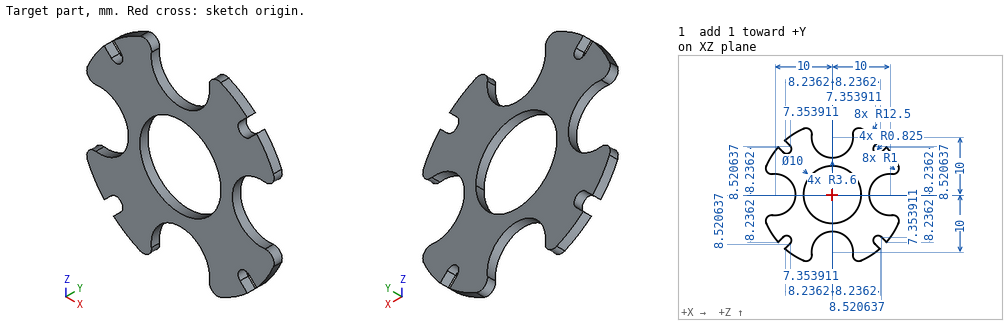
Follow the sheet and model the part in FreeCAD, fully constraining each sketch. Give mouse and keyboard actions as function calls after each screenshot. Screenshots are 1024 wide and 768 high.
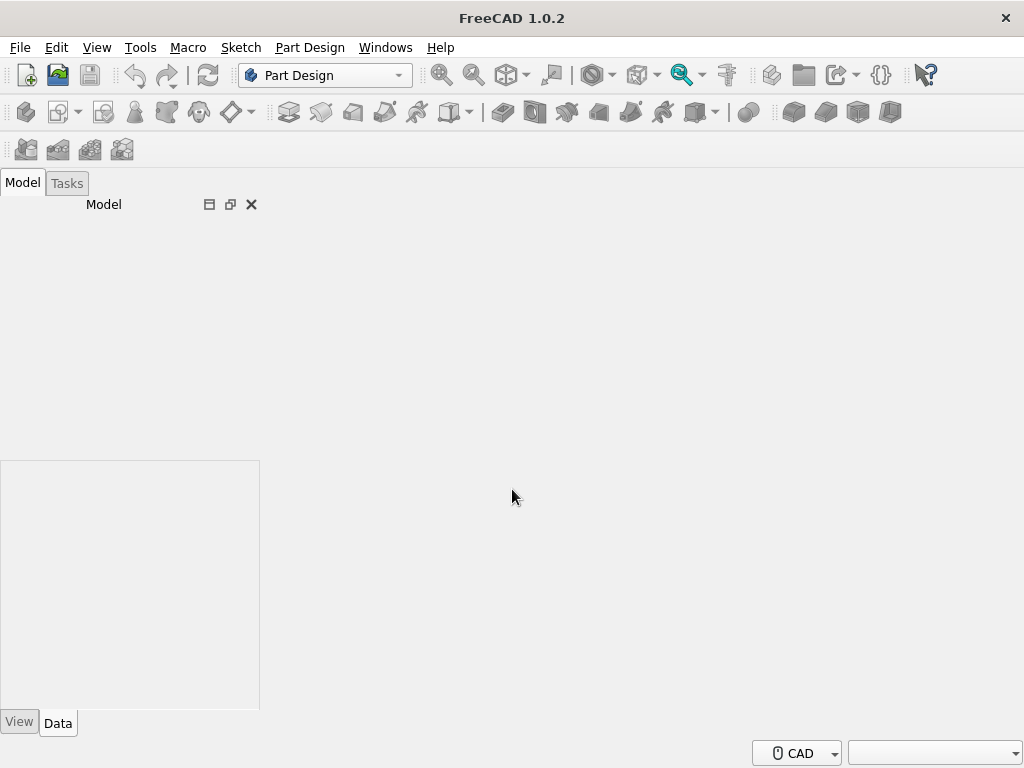
click(26, 76)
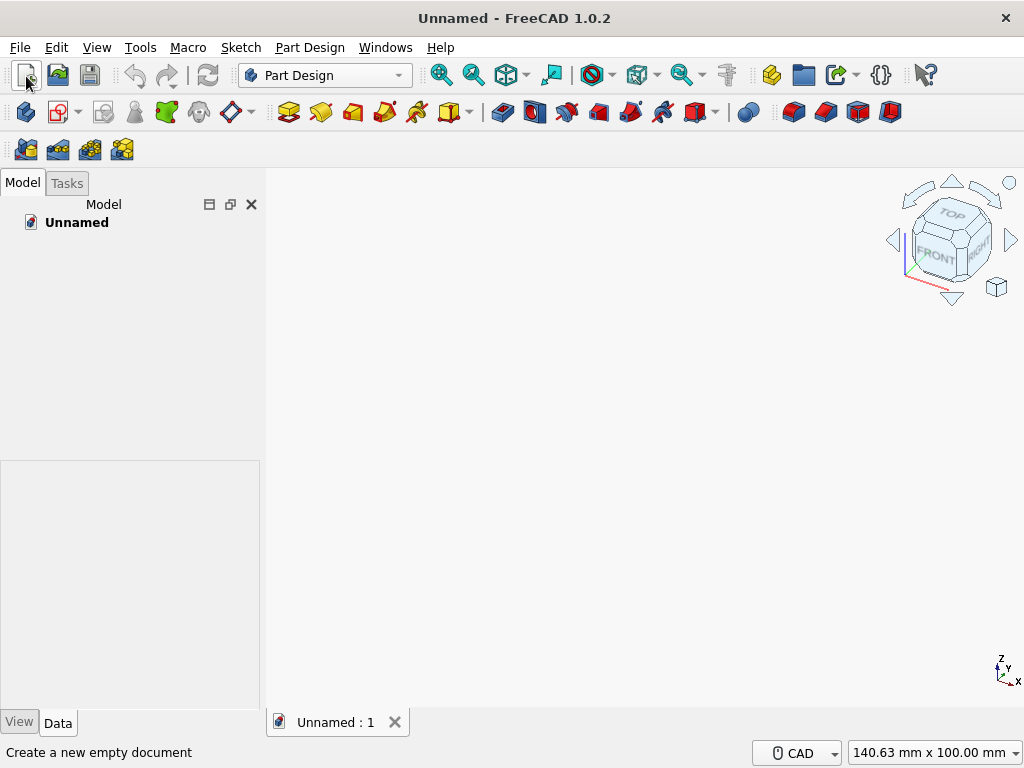
click(58, 112)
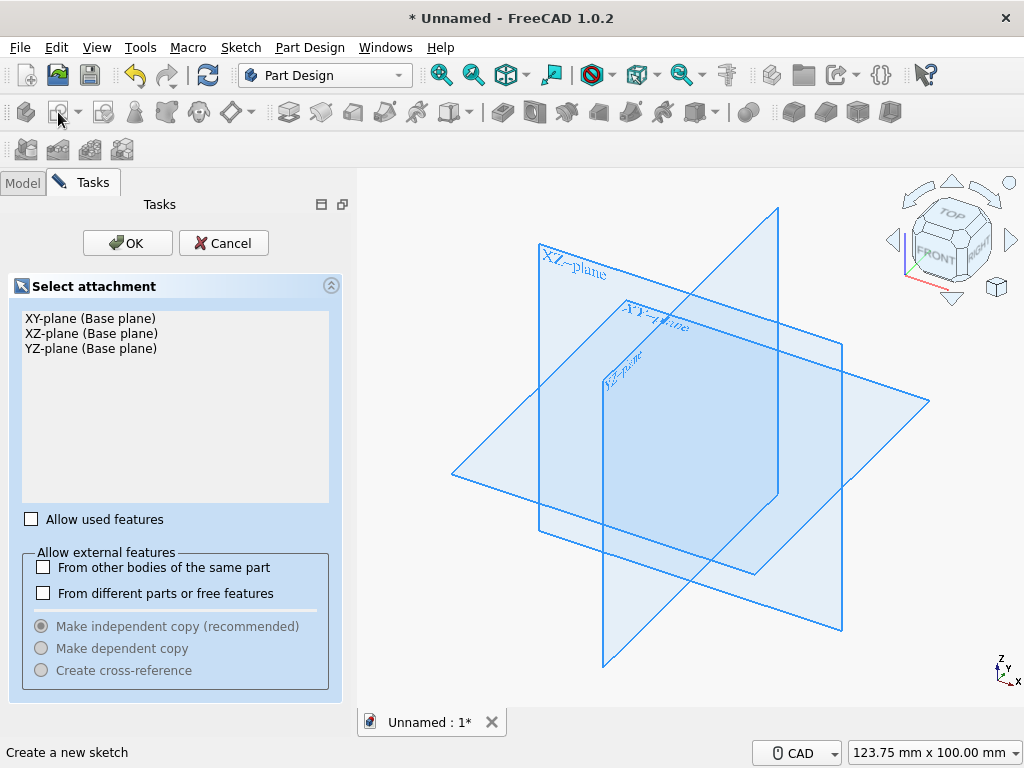
click(82, 334)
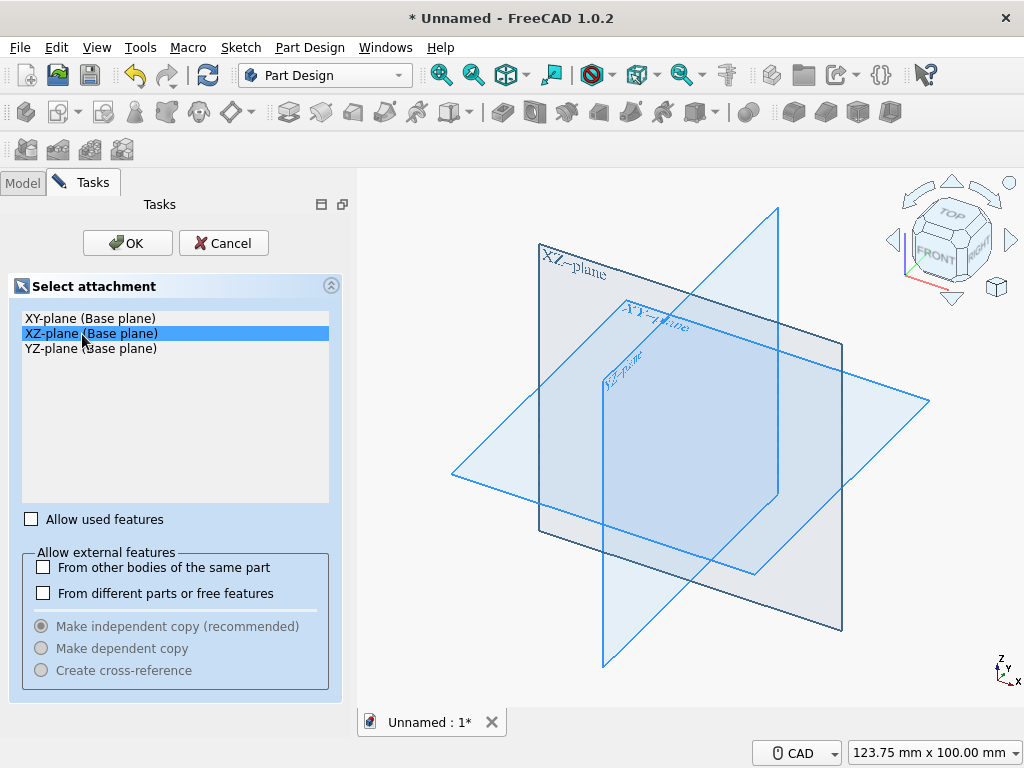
click(128, 243)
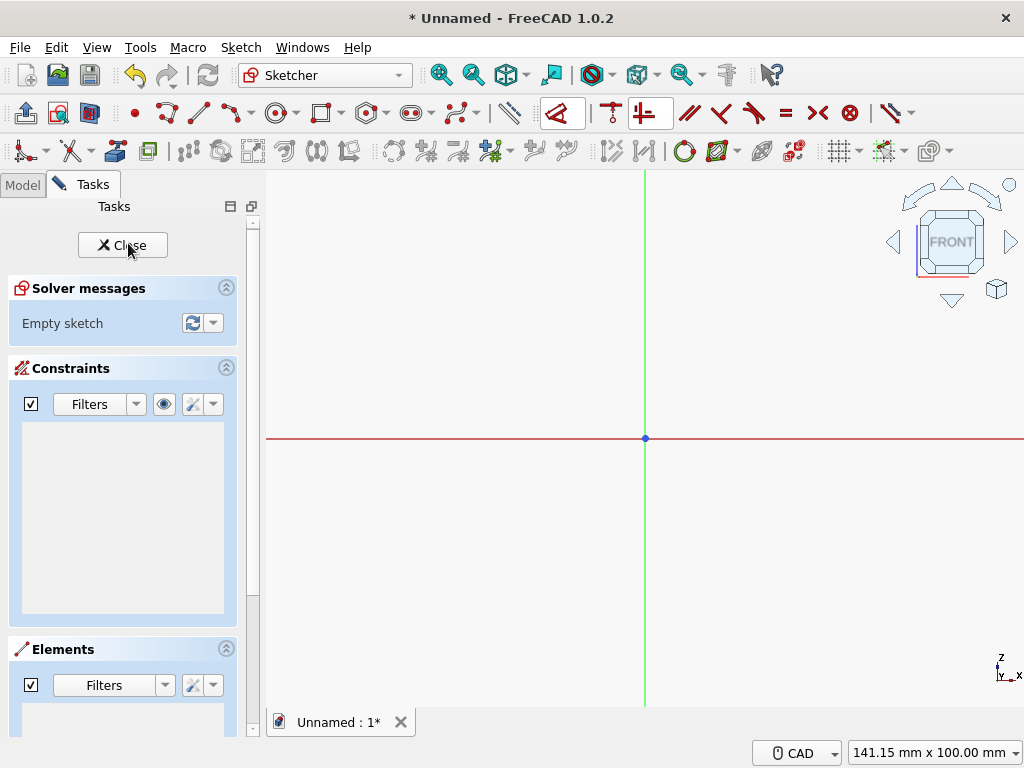
scroll(685, 439, up, 5)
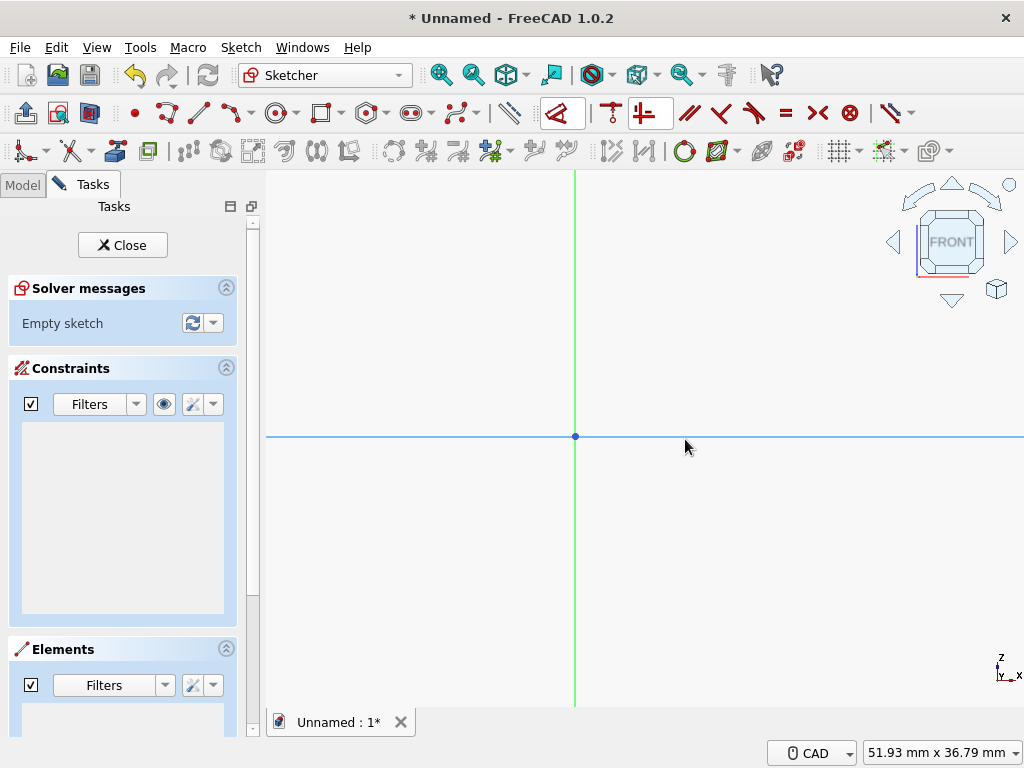
click(200, 114)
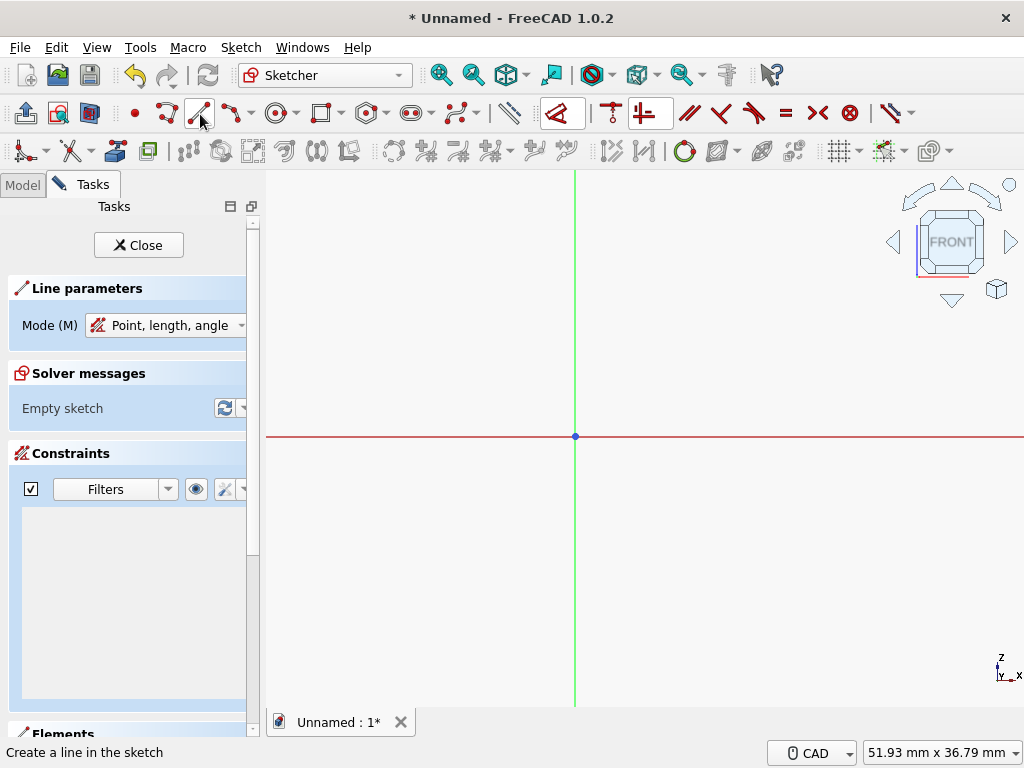
click(468, 312)
click(455, 300)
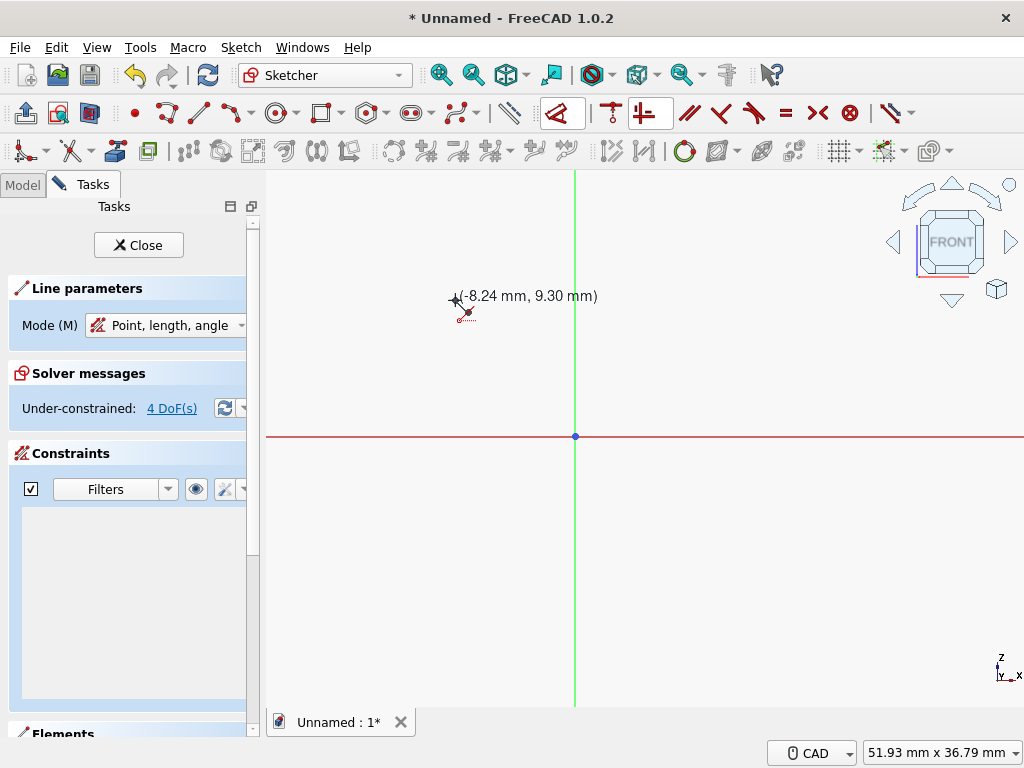
click(696, 300)
click(683, 312)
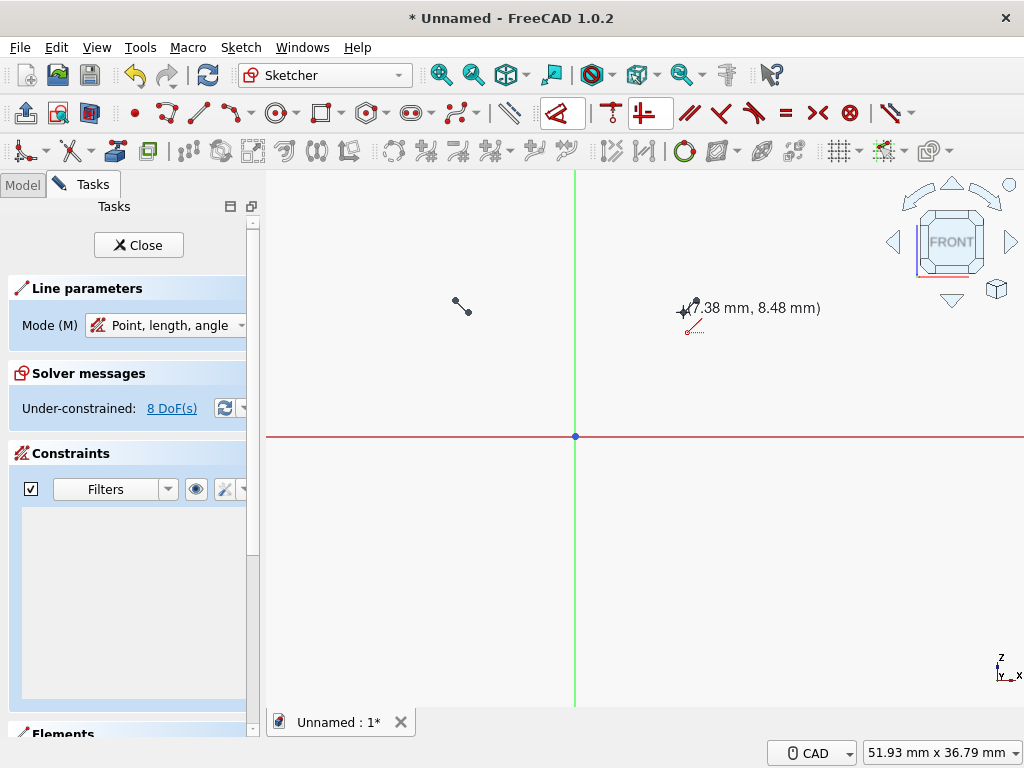
click(700, 329)
click(713, 317)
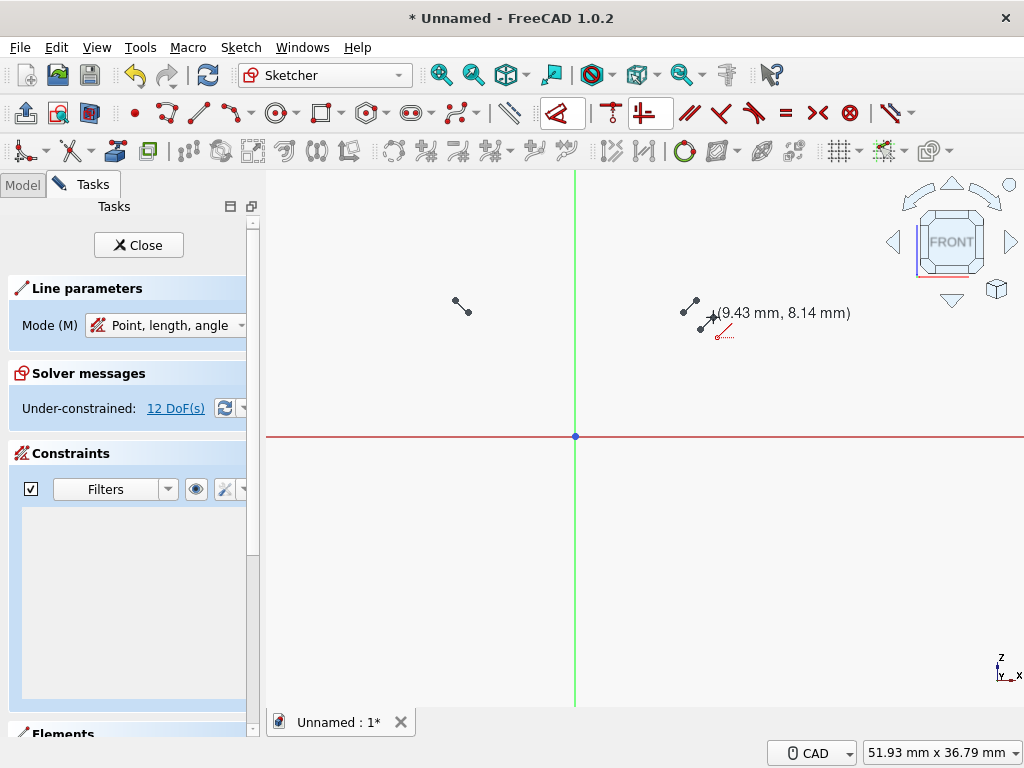
click(713, 557)
click(700, 544)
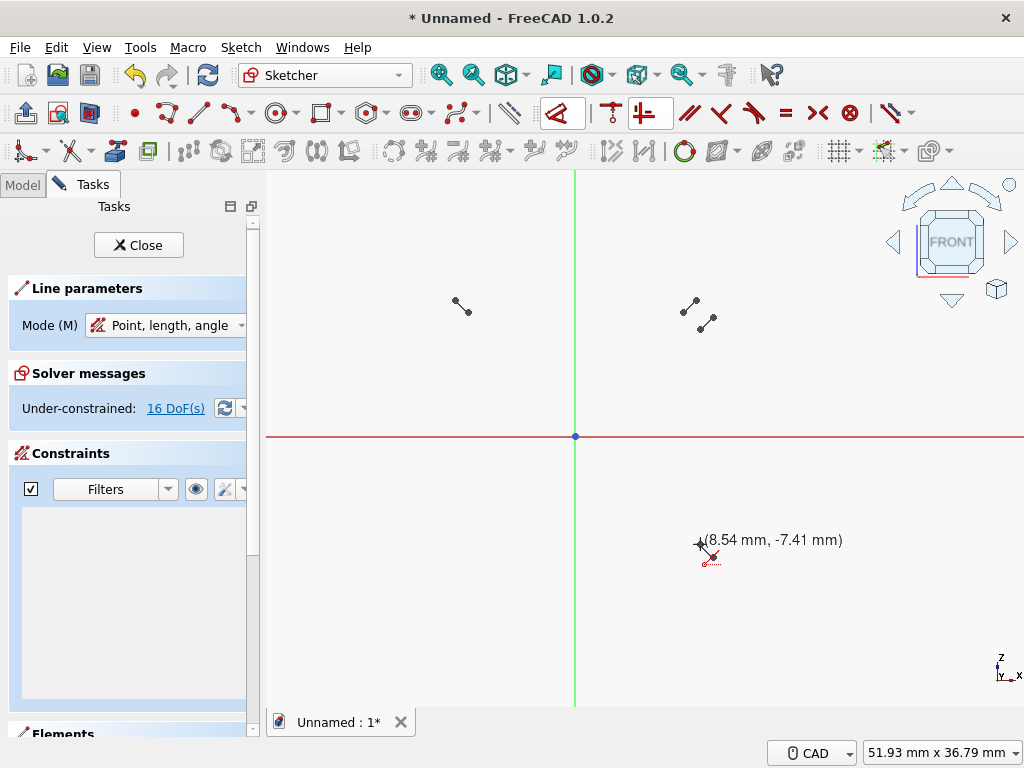
click(683, 561)
click(696, 574)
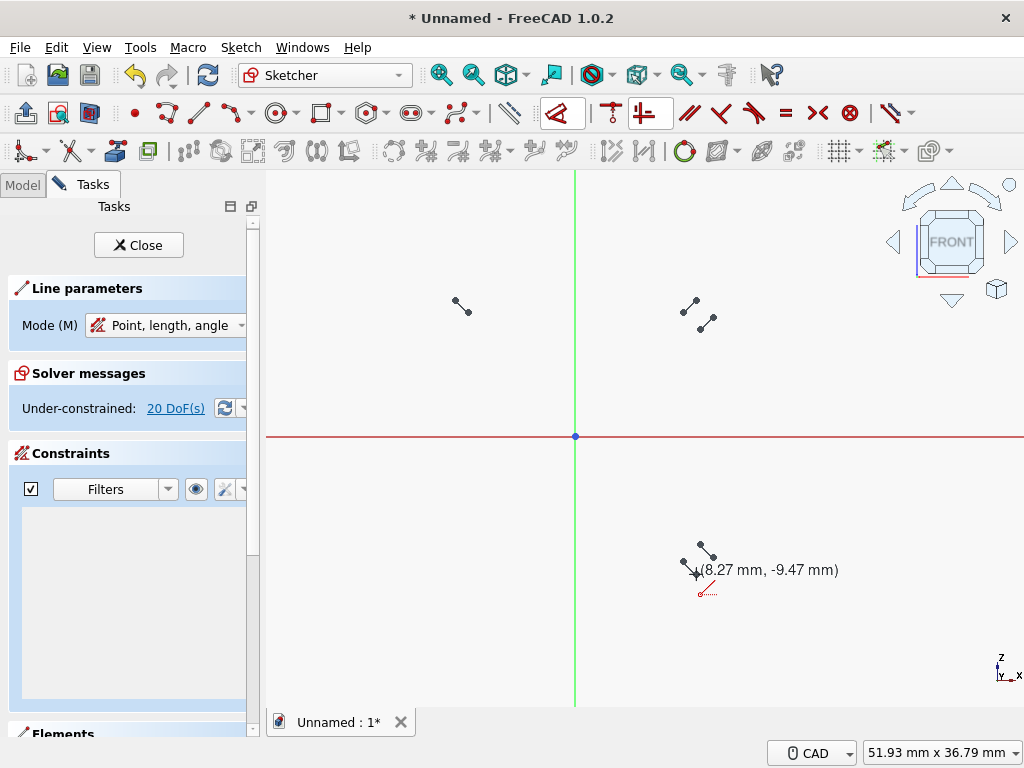
click(455, 574)
click(468, 561)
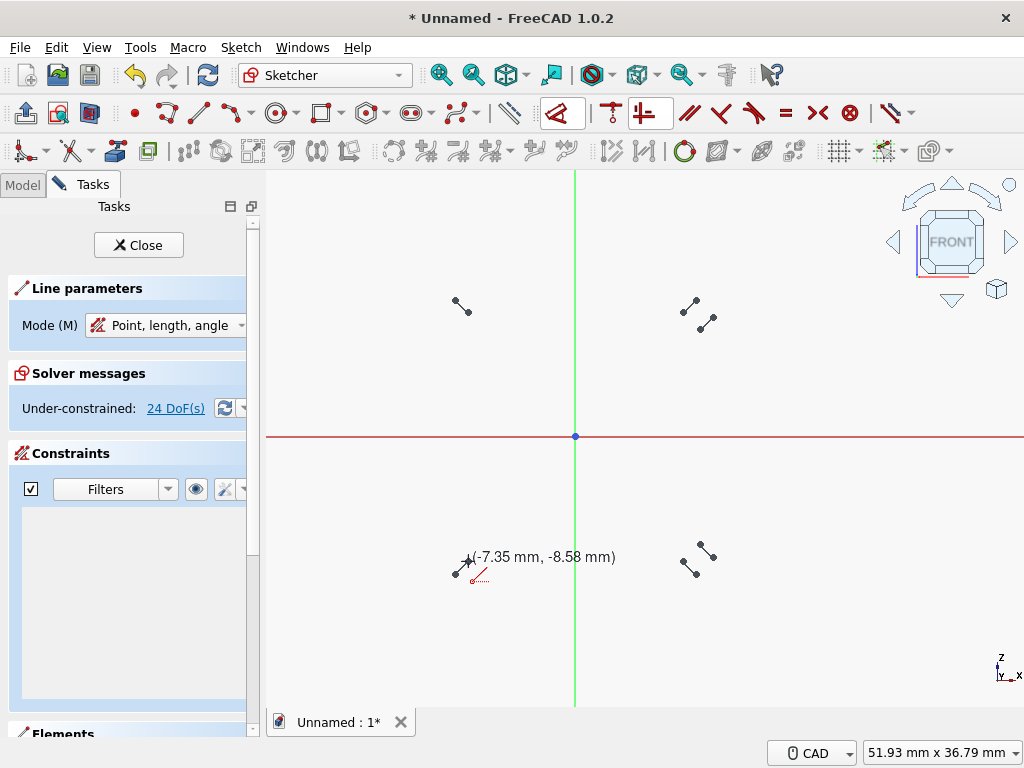
click(451, 544)
click(438, 557)